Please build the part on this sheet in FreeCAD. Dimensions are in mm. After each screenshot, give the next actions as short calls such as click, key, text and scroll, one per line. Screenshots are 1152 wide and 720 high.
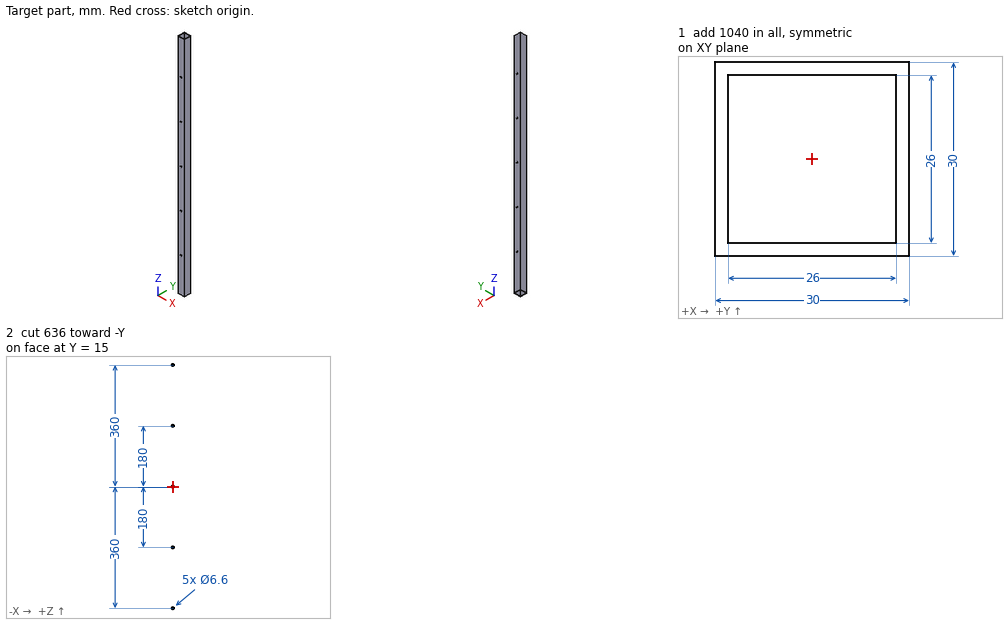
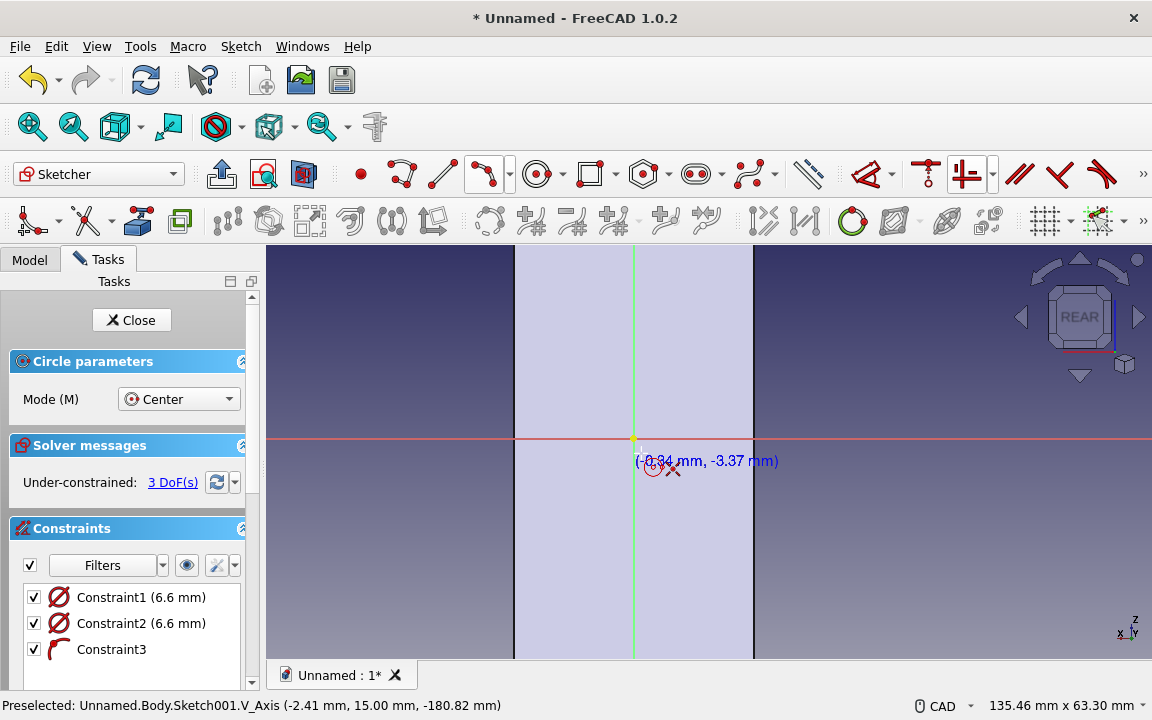
scroll(641, 453, down, 15)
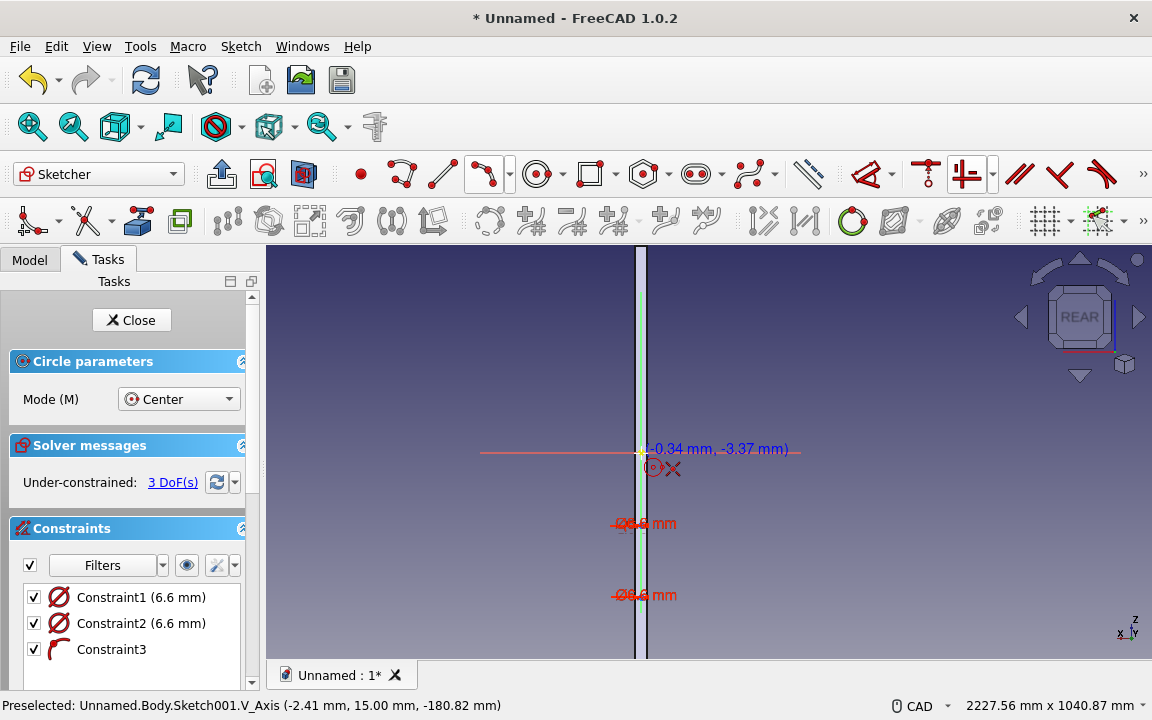
click(641, 453)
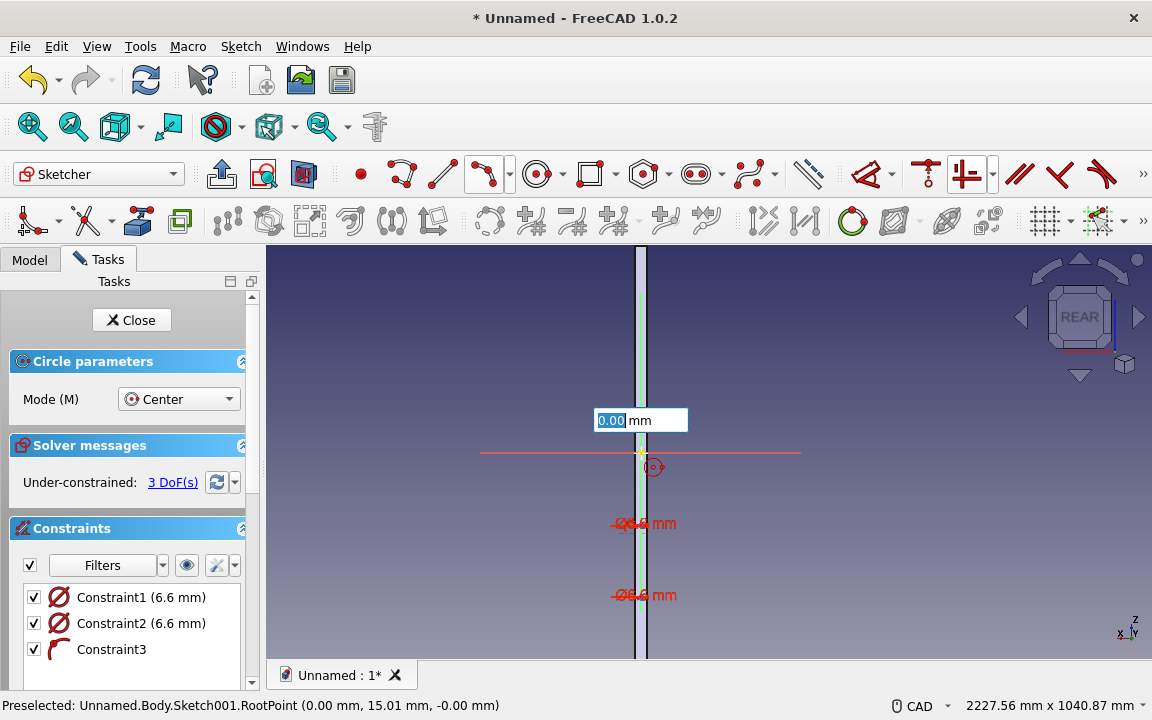
scroll(642, 452, up, 15)
move(633, 439)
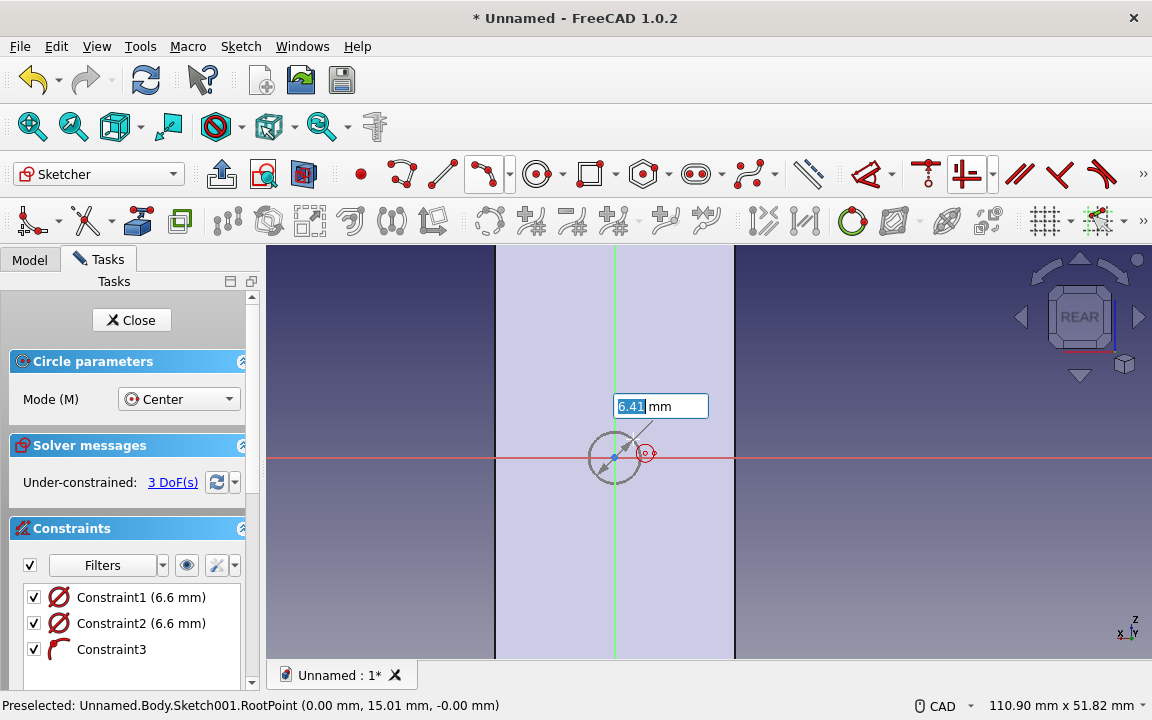
text(6.6)
key(Return)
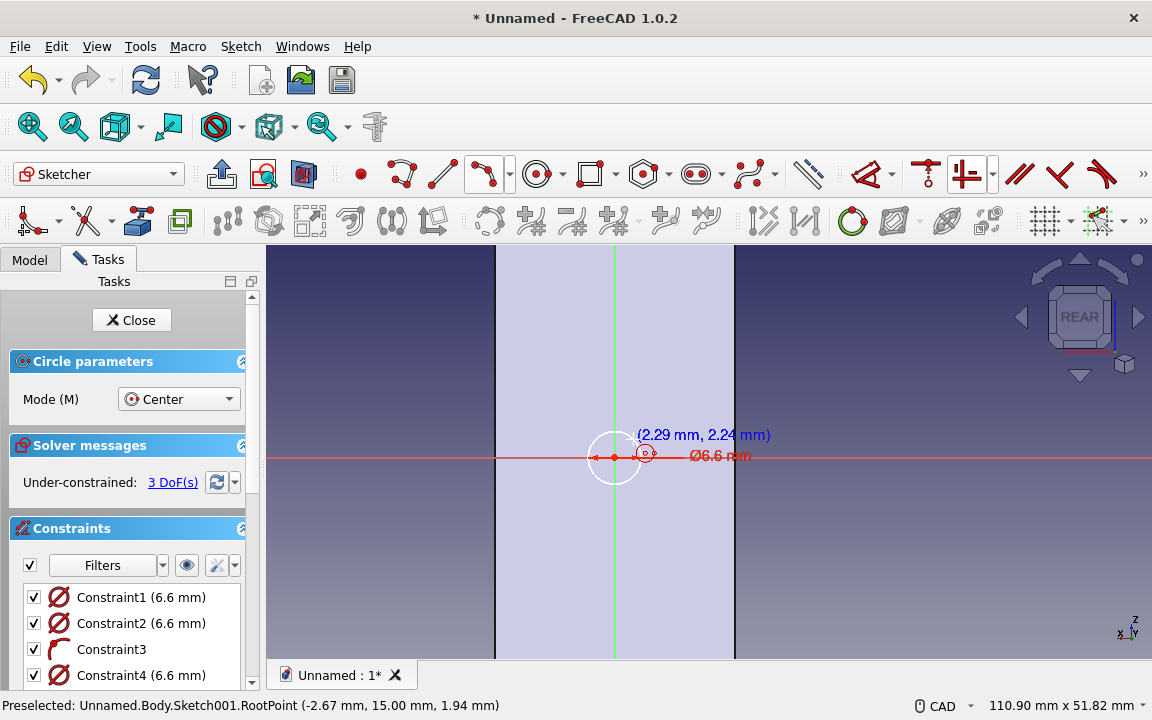
scroll(642, 452, down, 15)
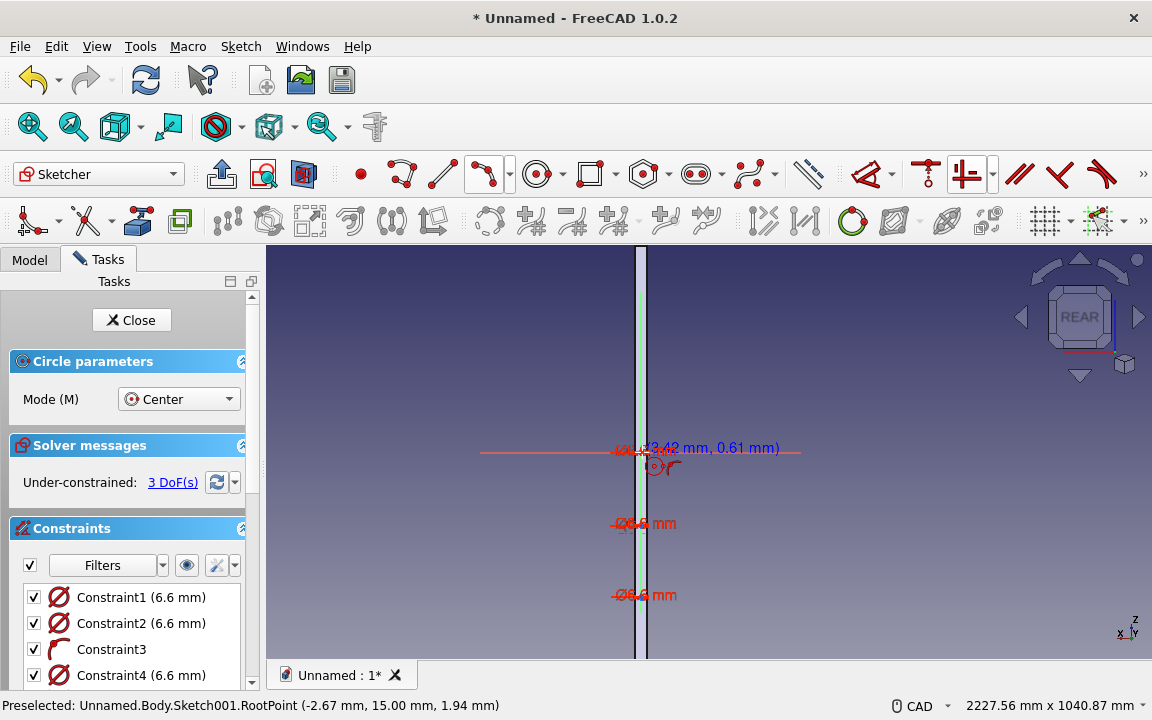
scroll(641, 381, up, 15)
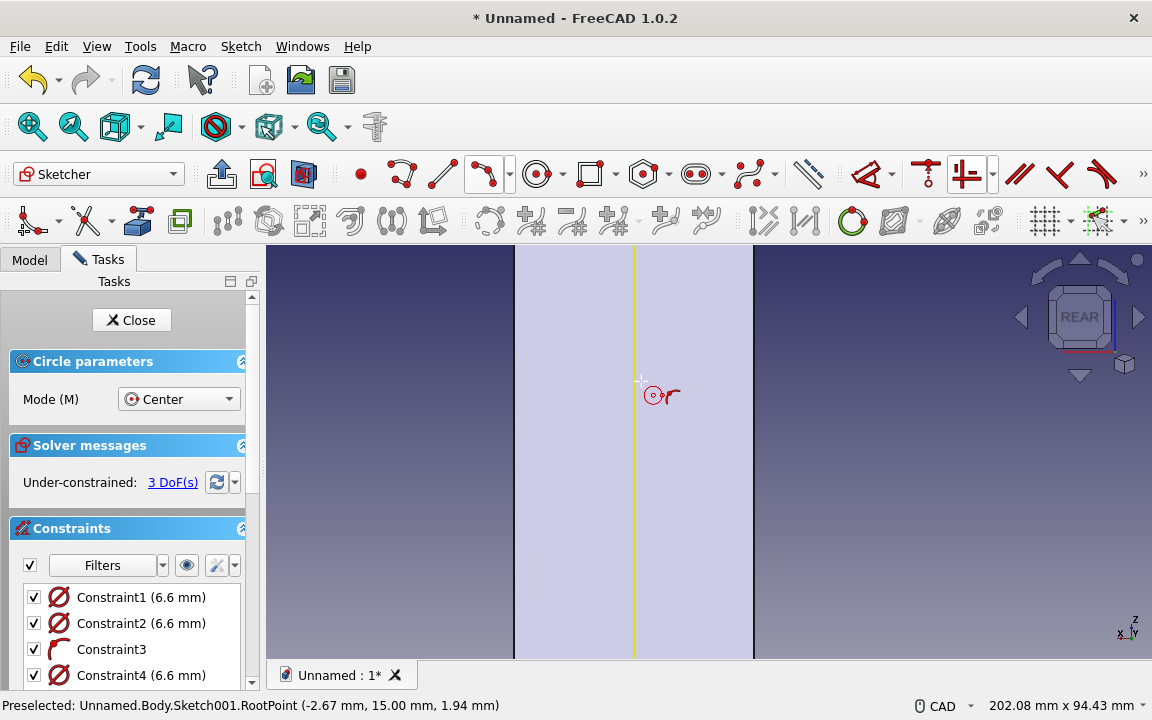
scroll(641, 381, down, 15)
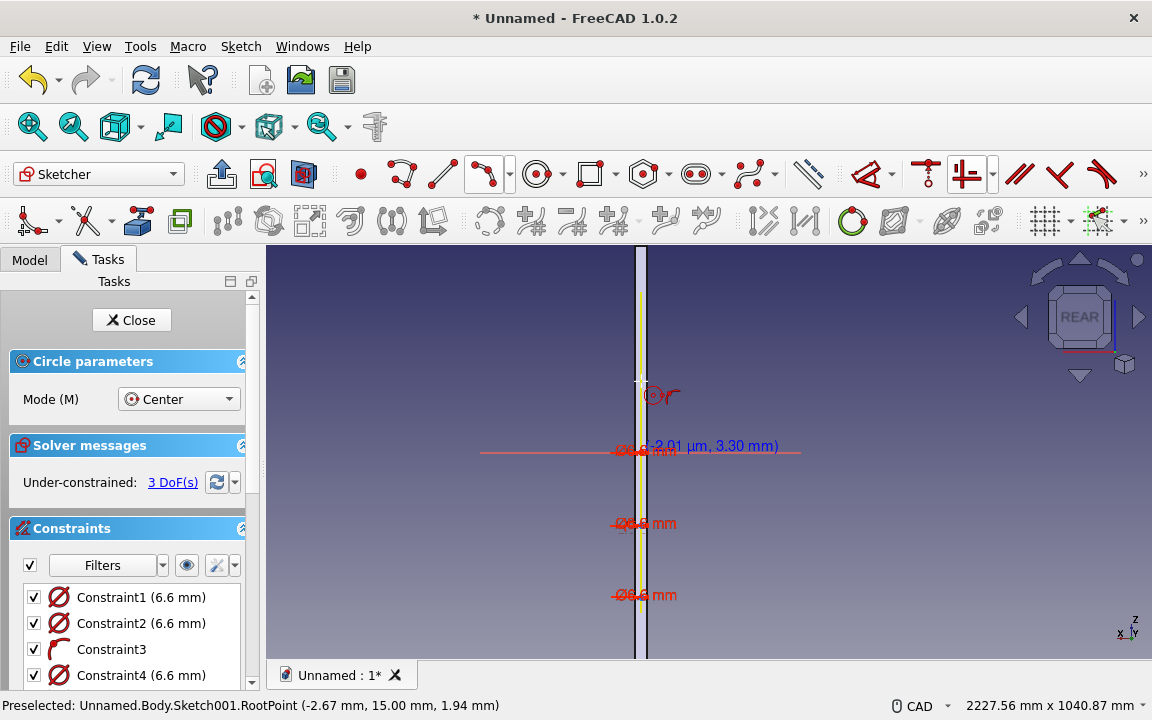
click(641, 381)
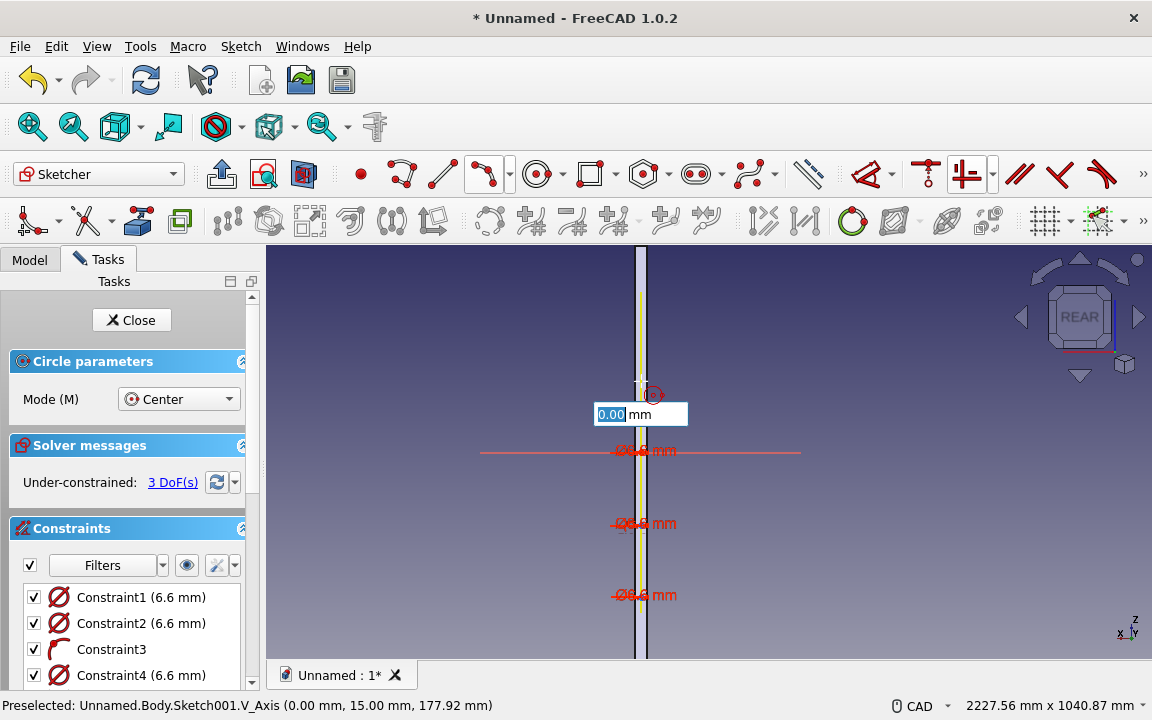
scroll(642, 381, up, 13)
move(640, 373)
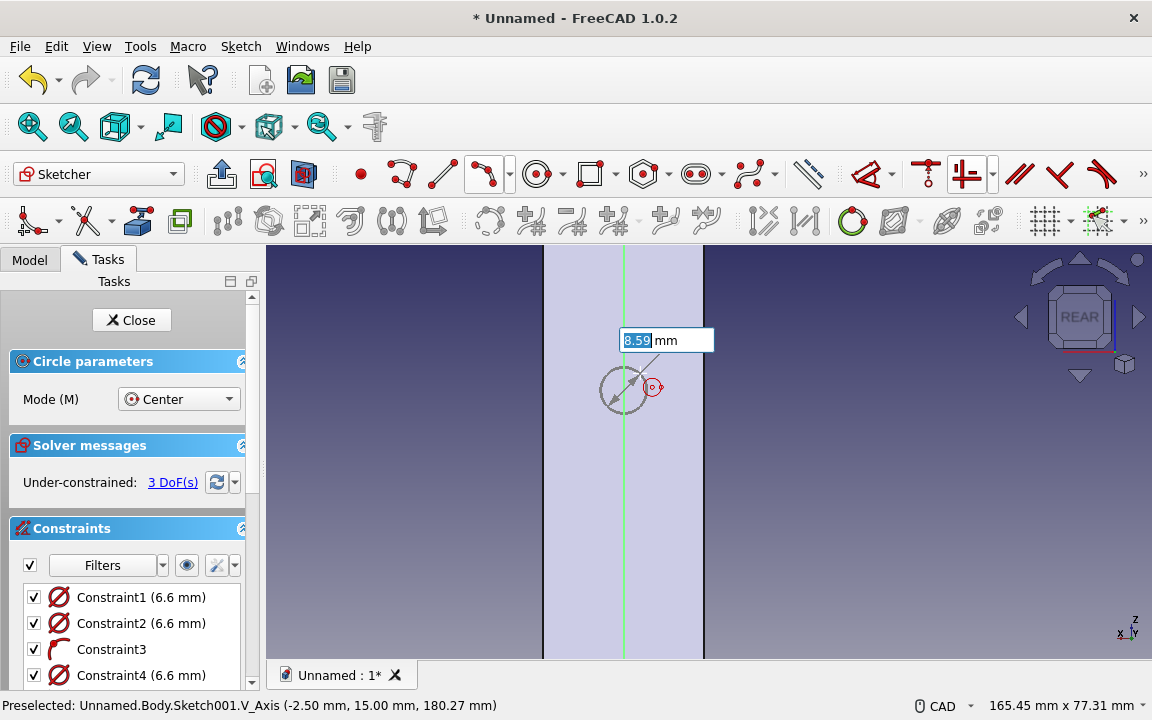
text(6.6)
key(Return)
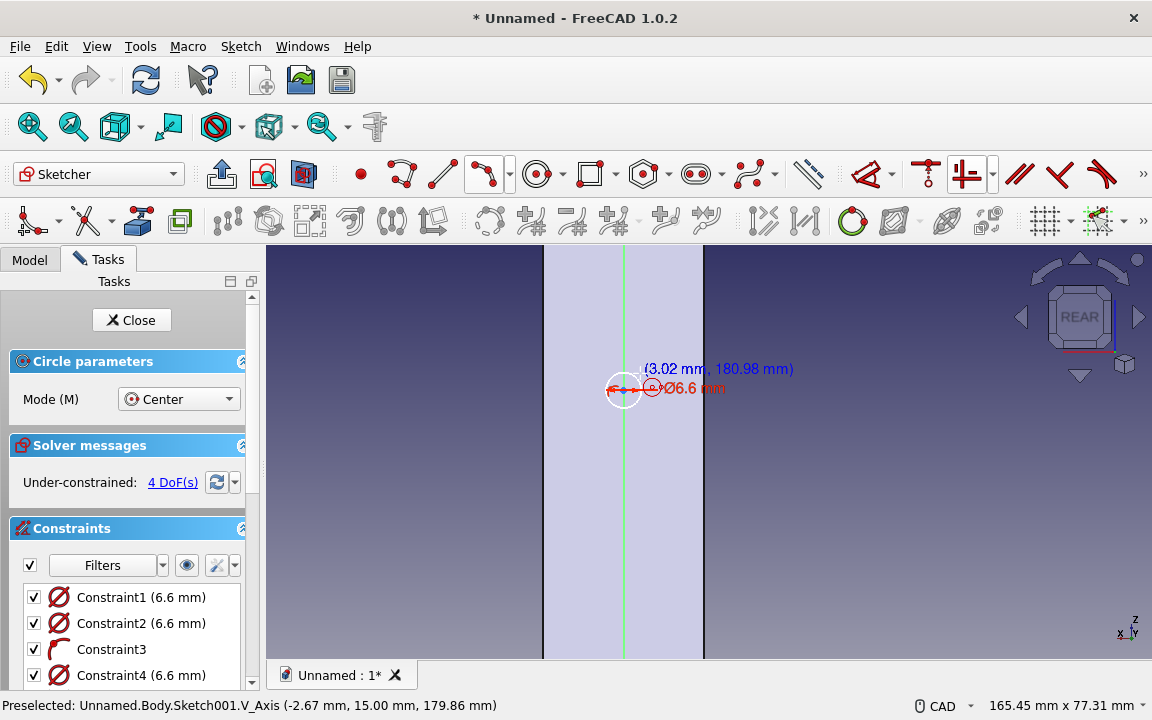
scroll(642, 394, down, 14)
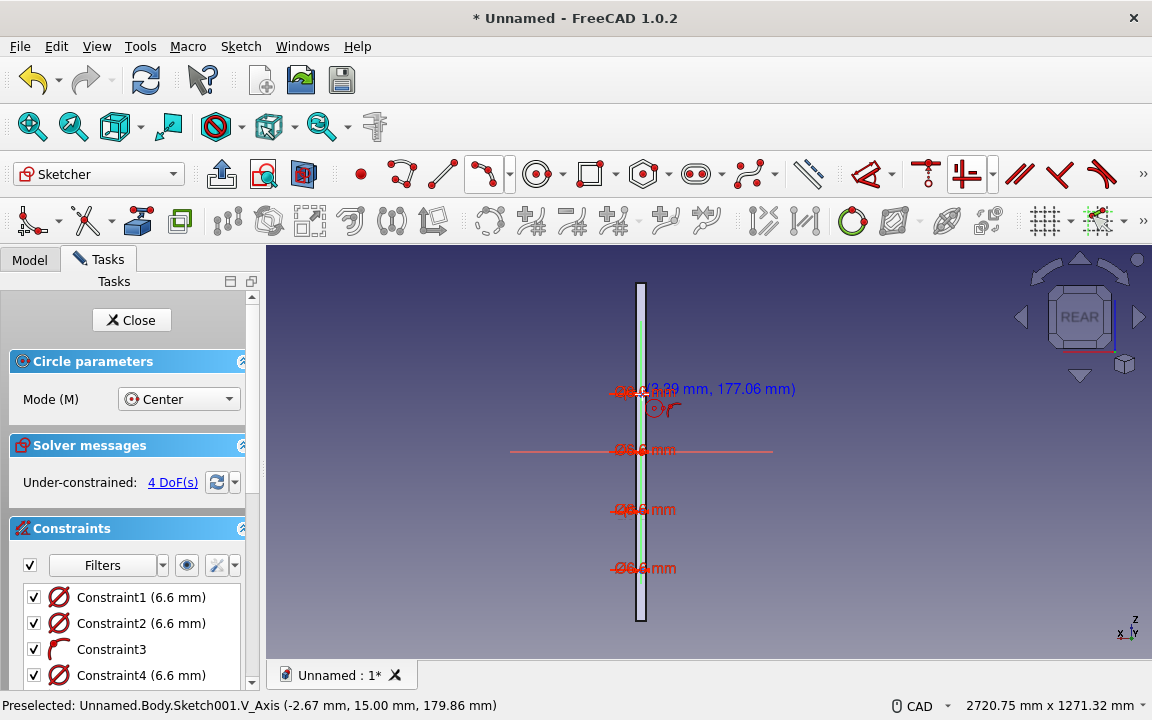
scroll(641, 335, up, 16)